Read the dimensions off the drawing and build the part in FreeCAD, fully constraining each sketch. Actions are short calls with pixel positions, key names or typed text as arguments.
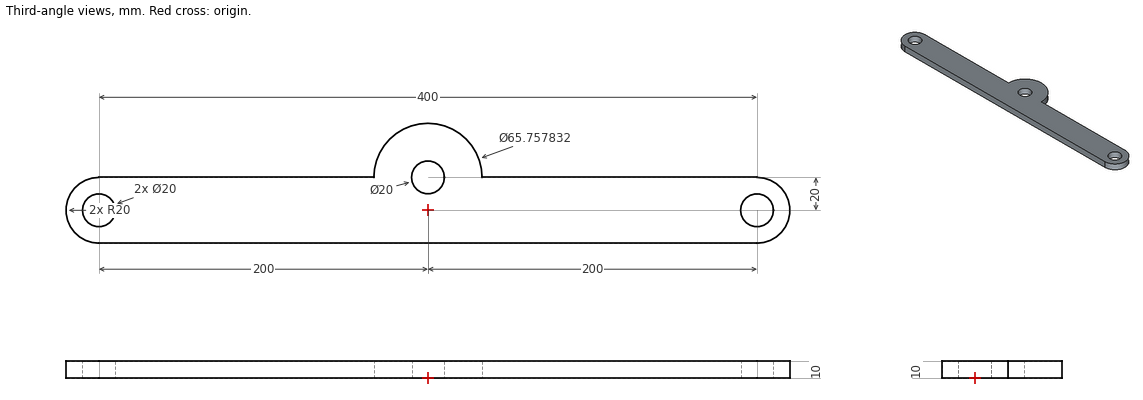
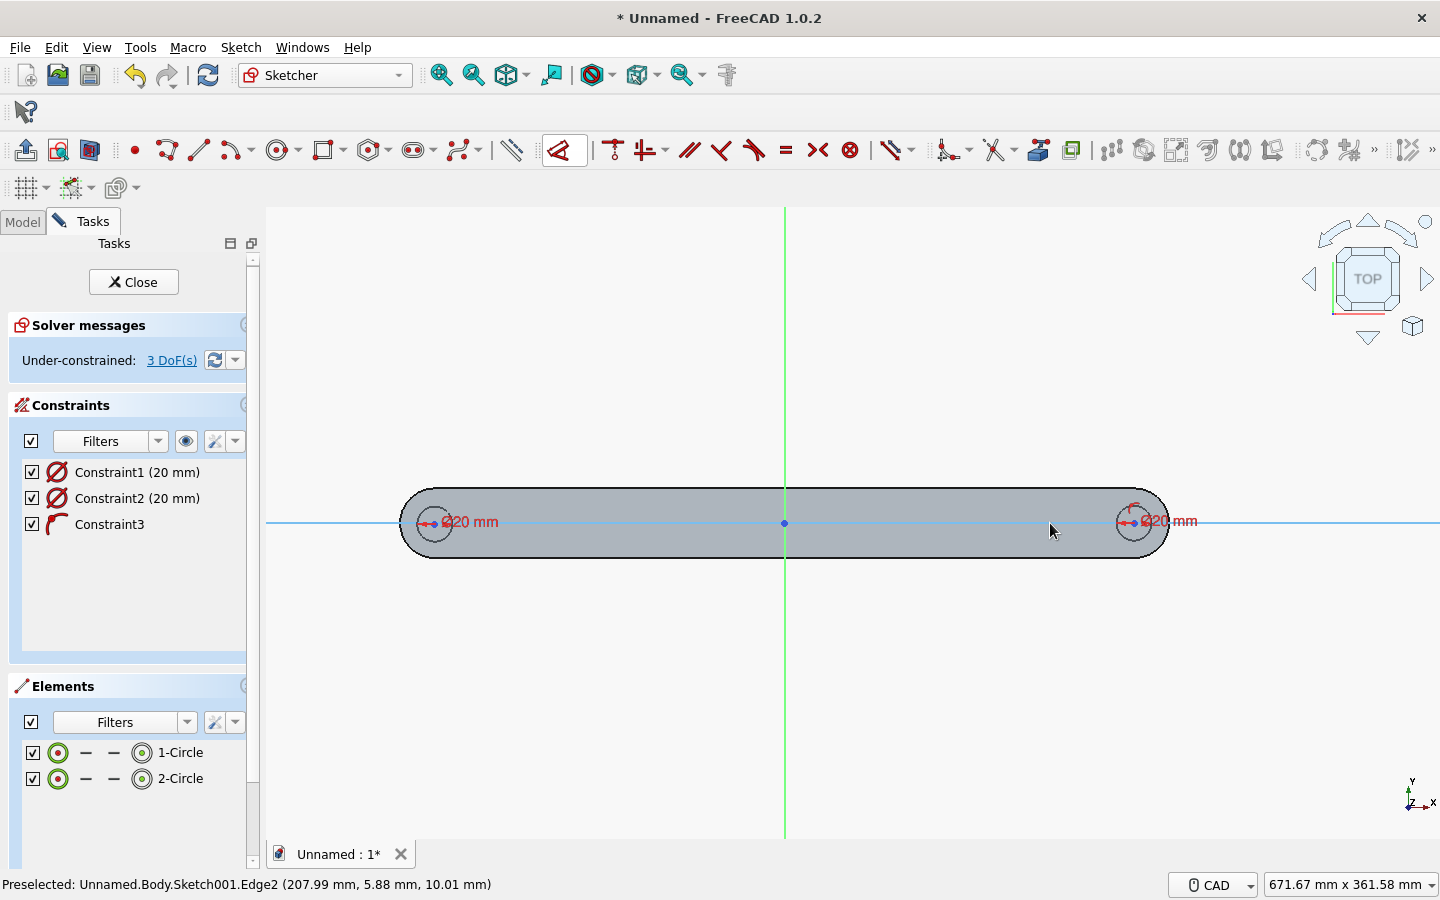
click(435, 524)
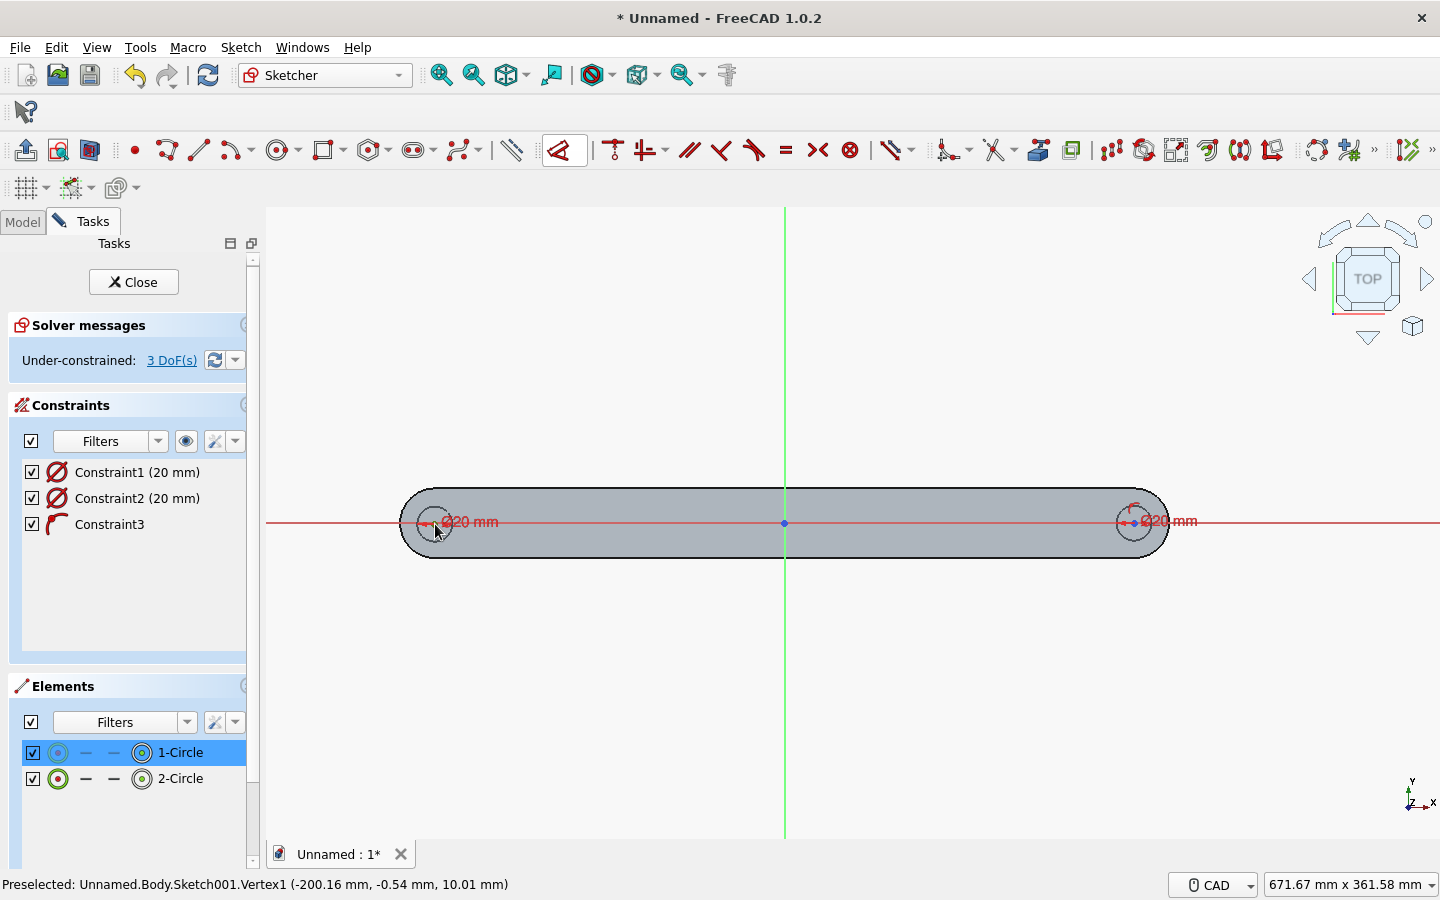
click(364, 523)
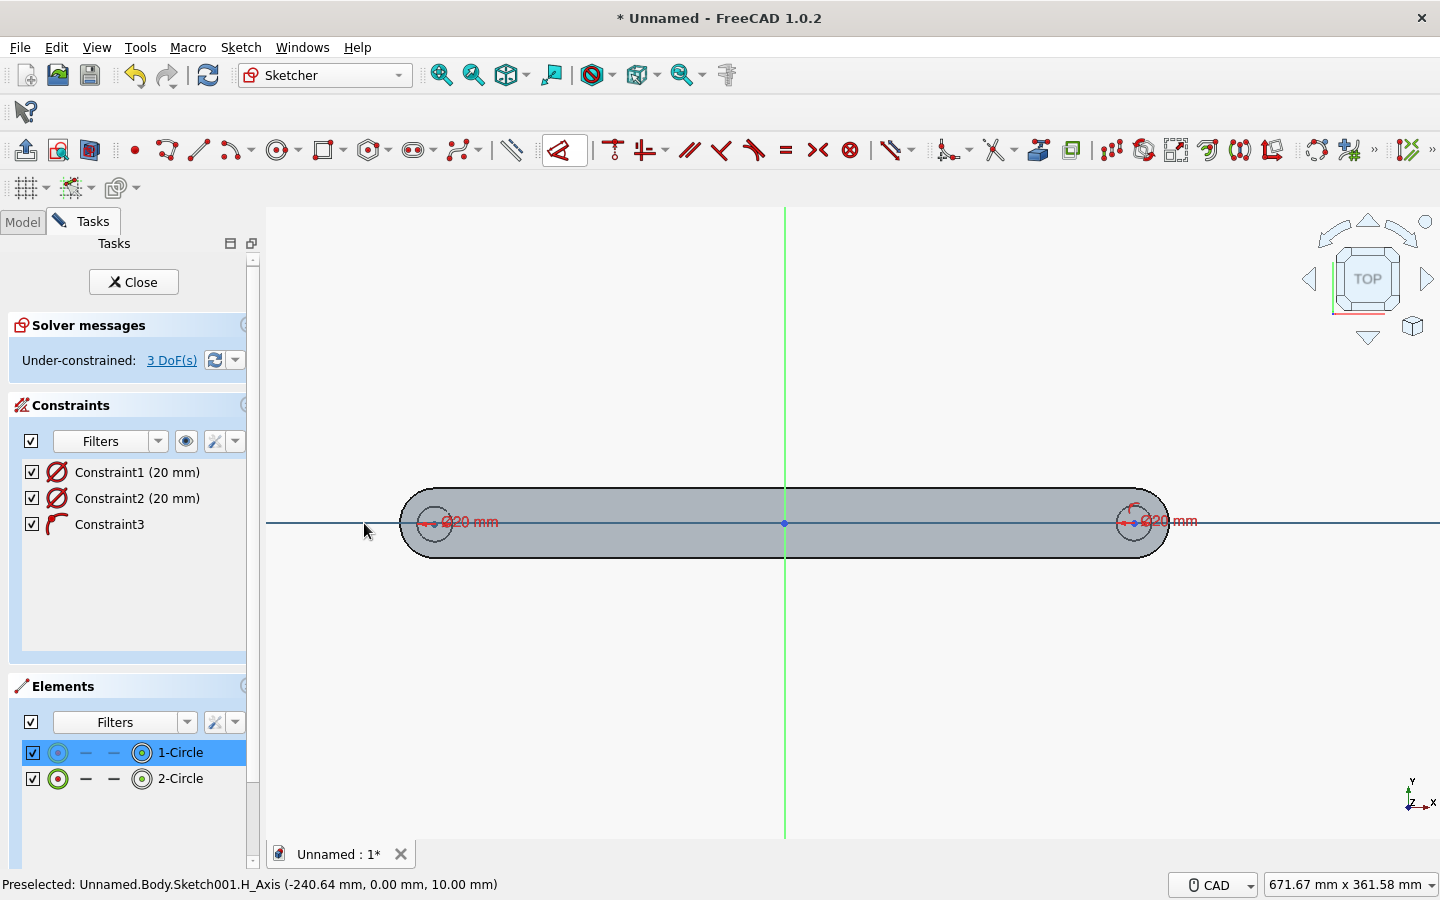
click(614, 150)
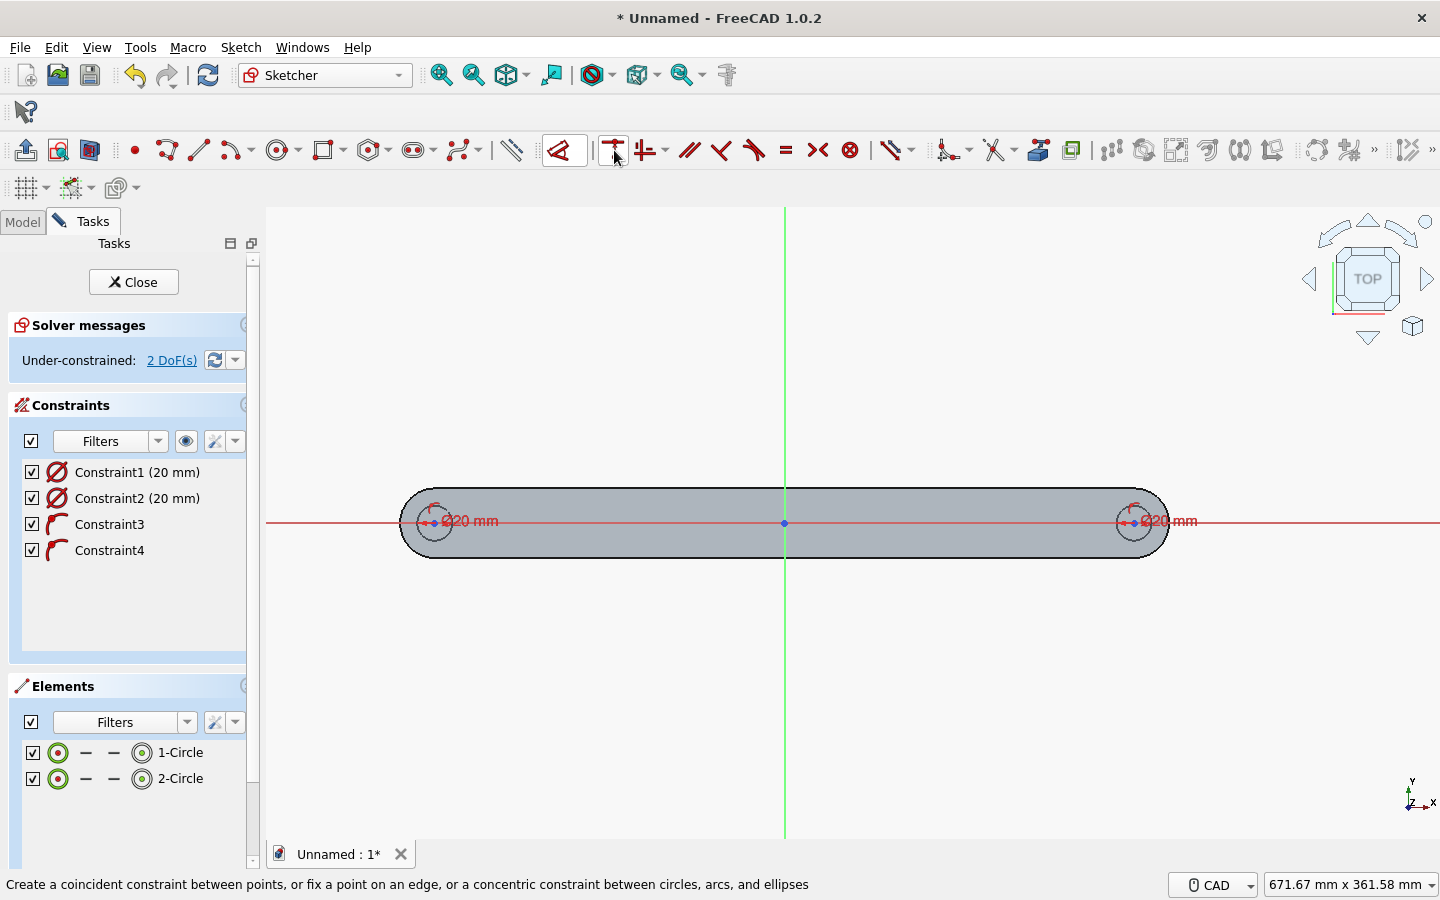
click(435, 523)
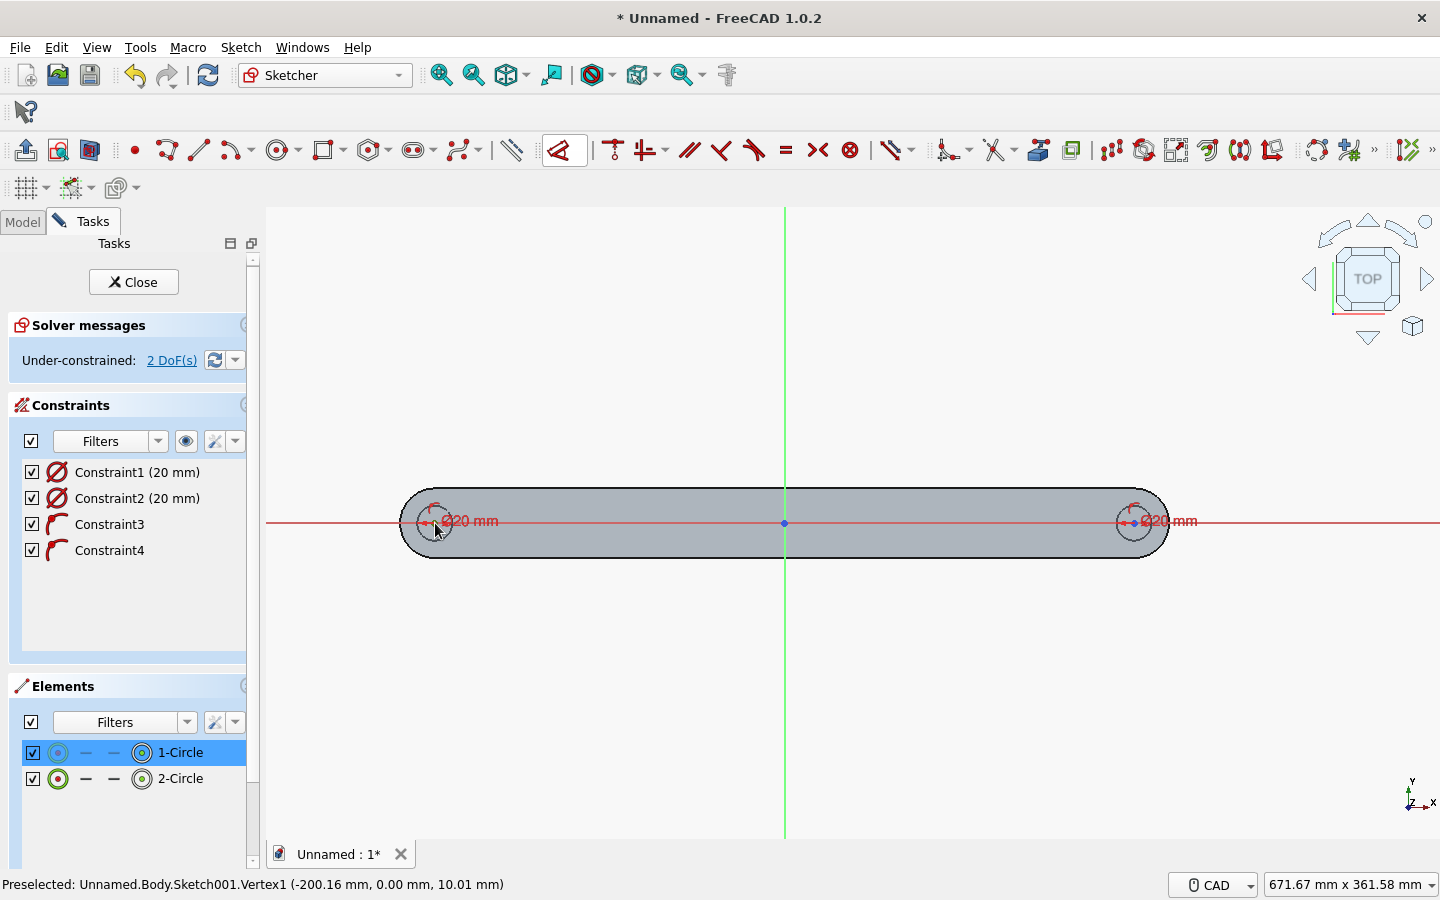
click(582, 150)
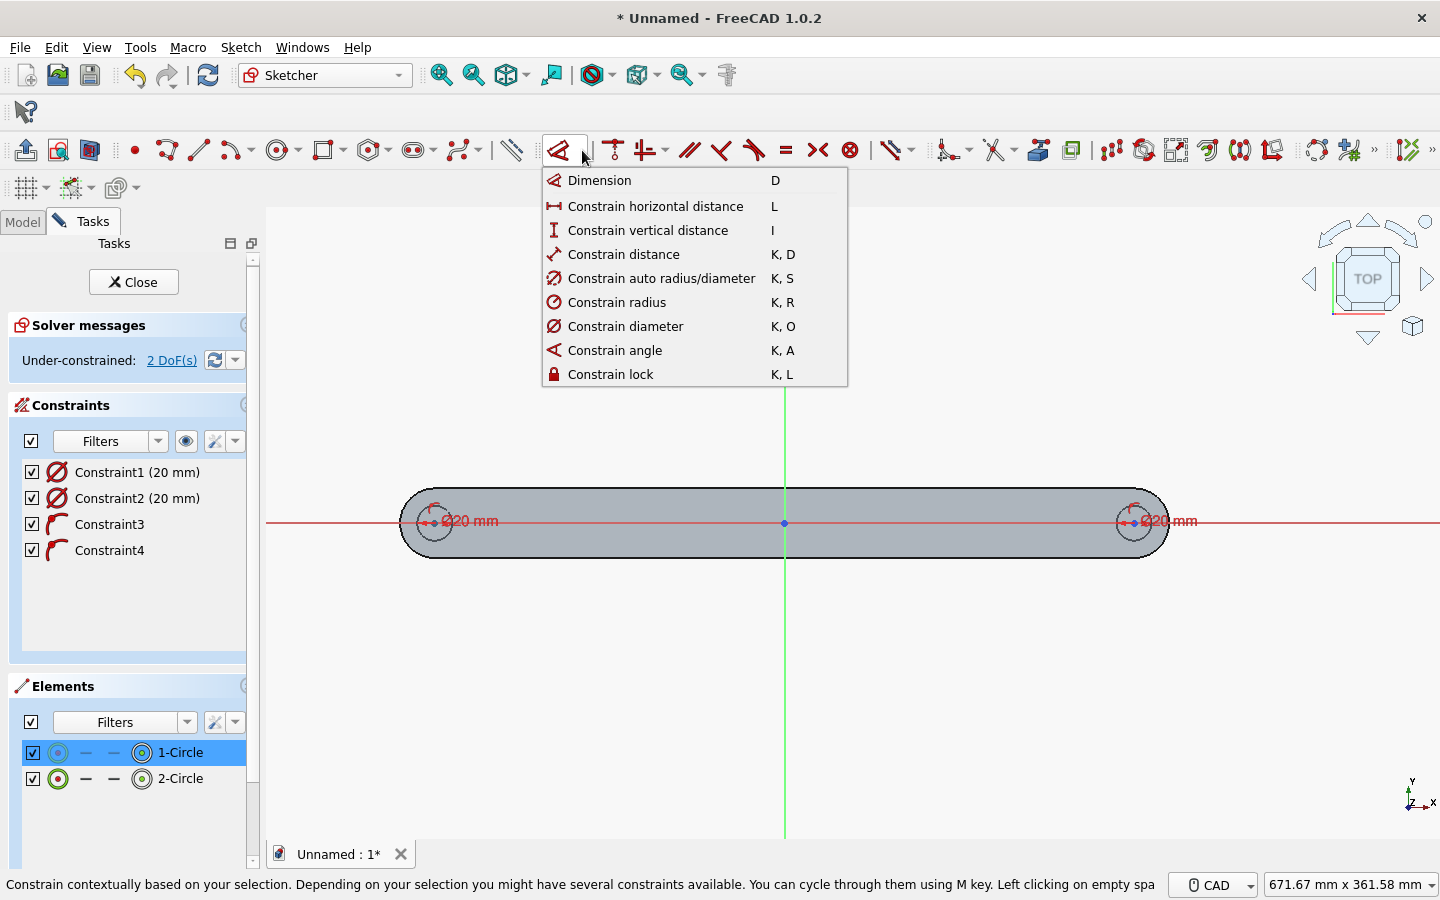
click(695, 206)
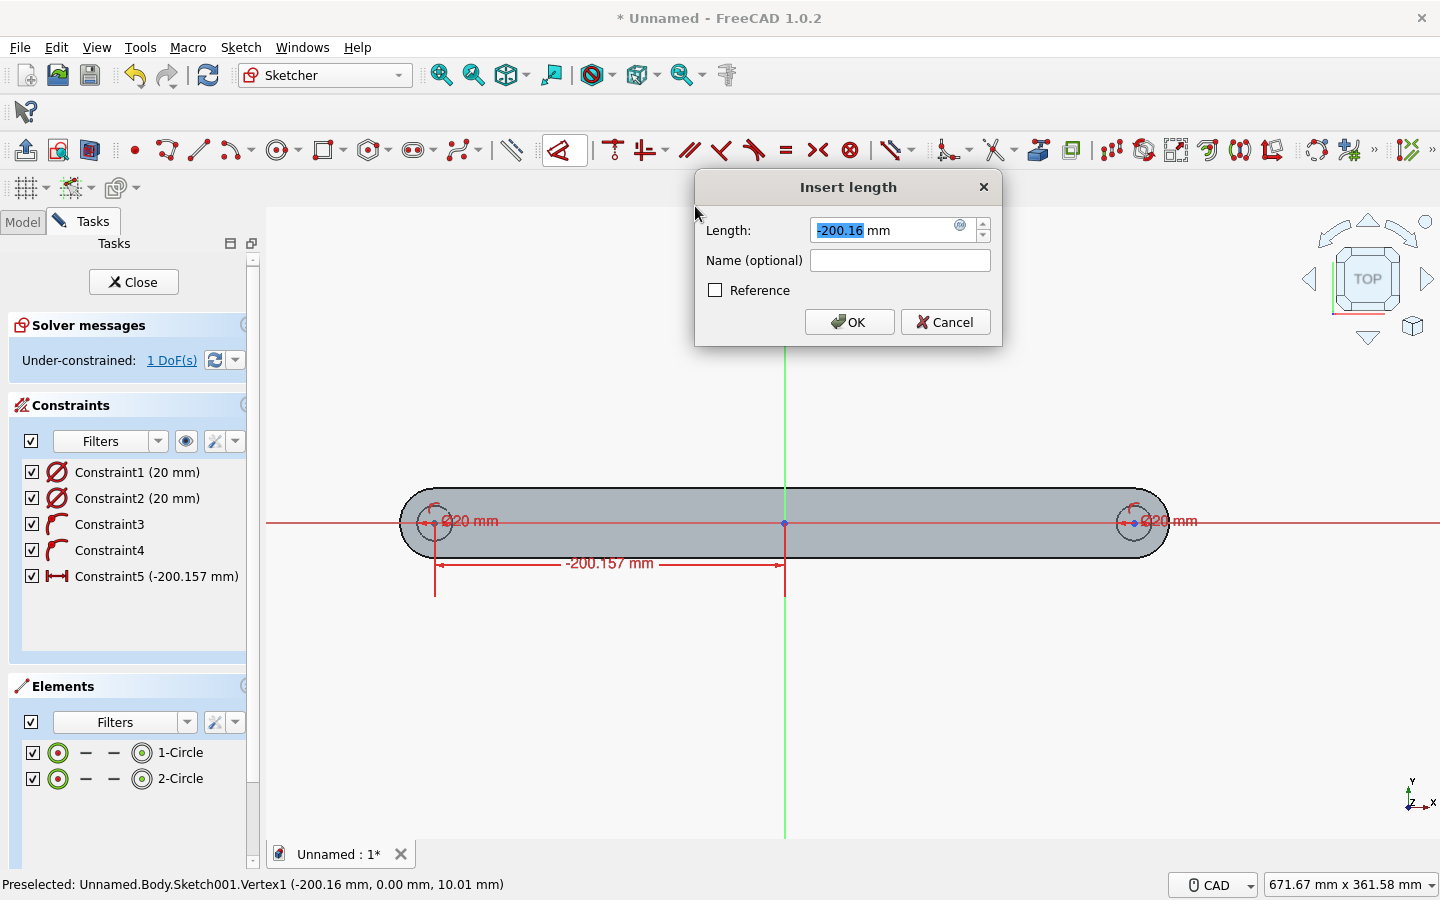
text(-200)
key(Return)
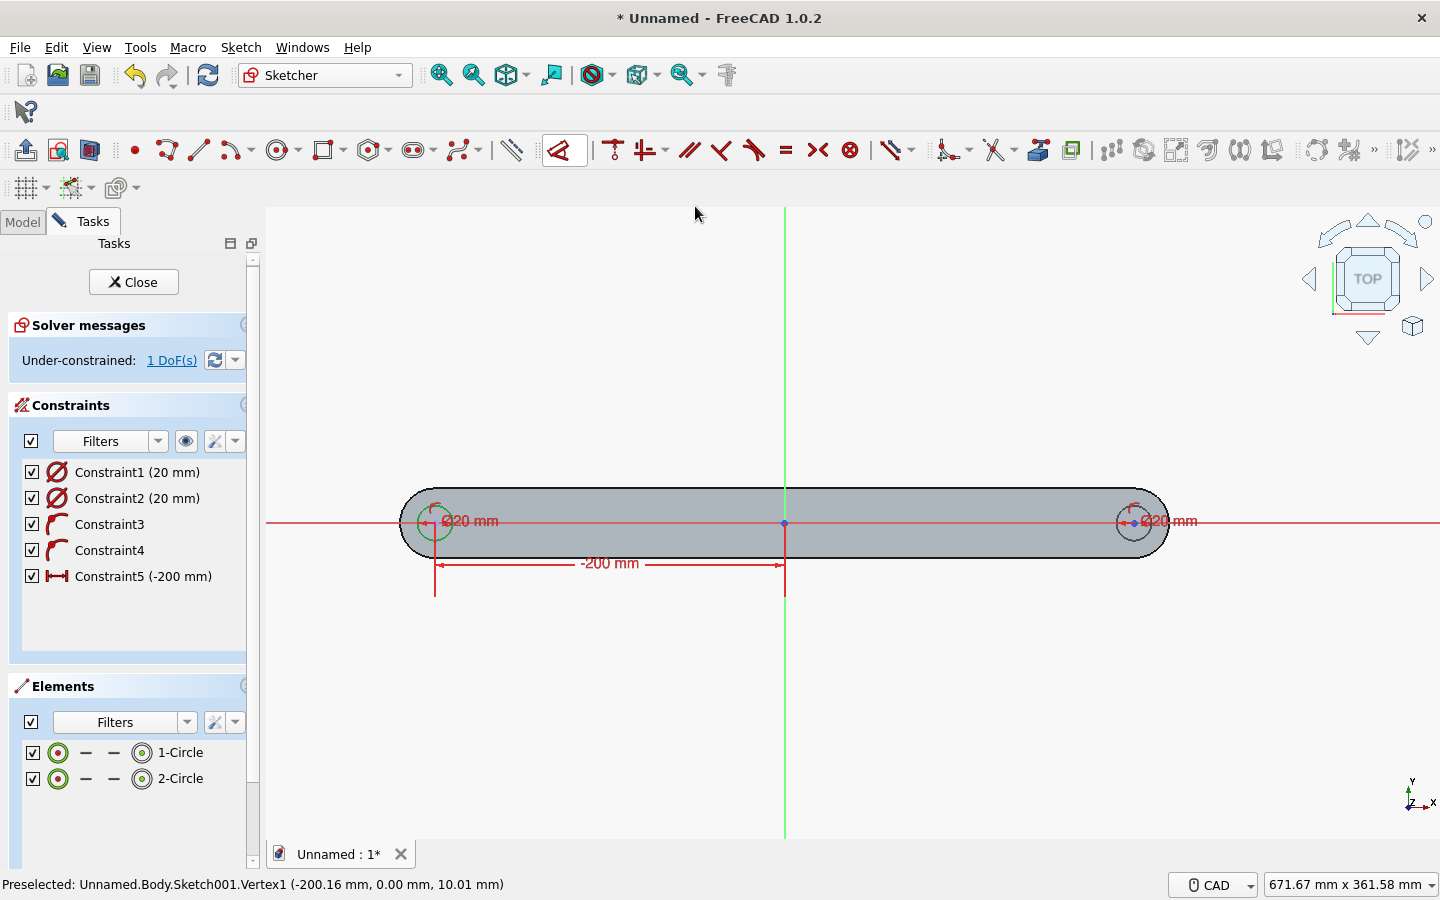
click(1134, 523)